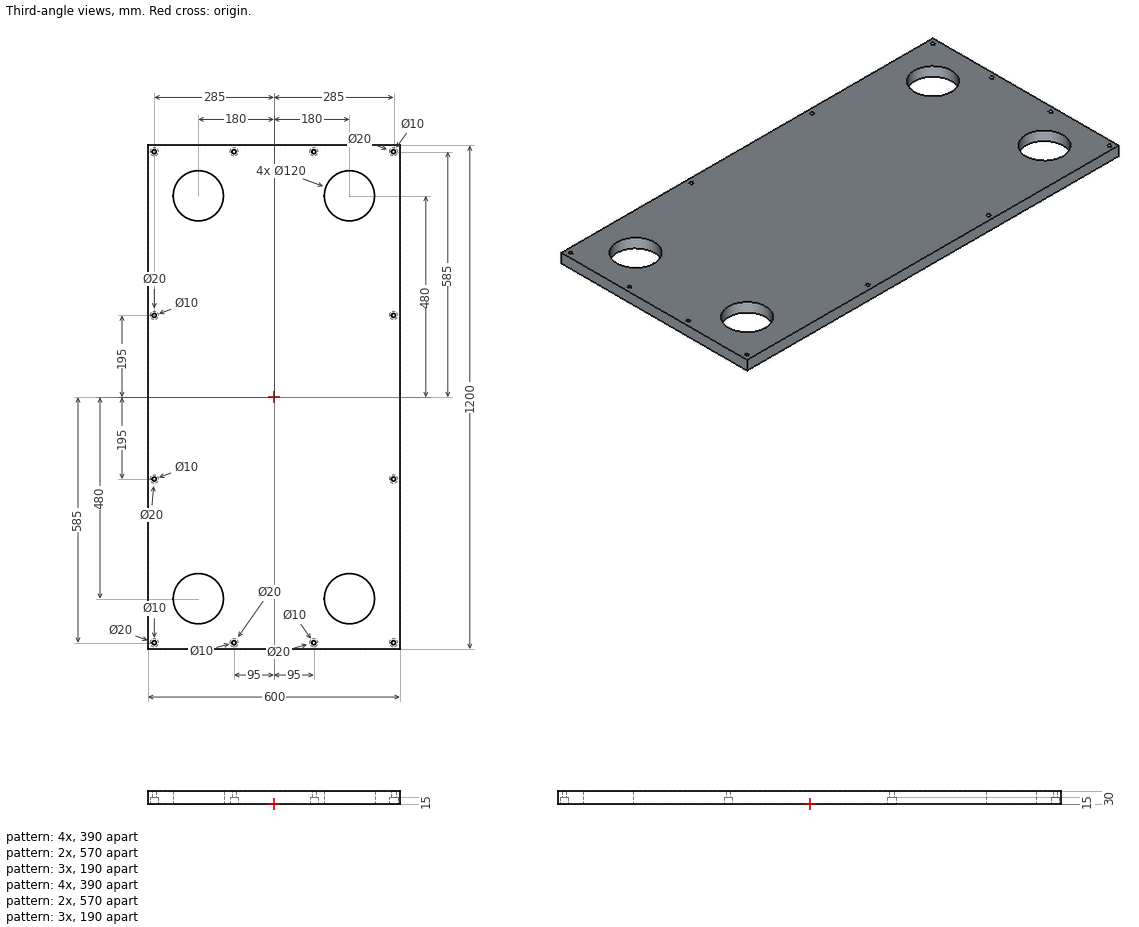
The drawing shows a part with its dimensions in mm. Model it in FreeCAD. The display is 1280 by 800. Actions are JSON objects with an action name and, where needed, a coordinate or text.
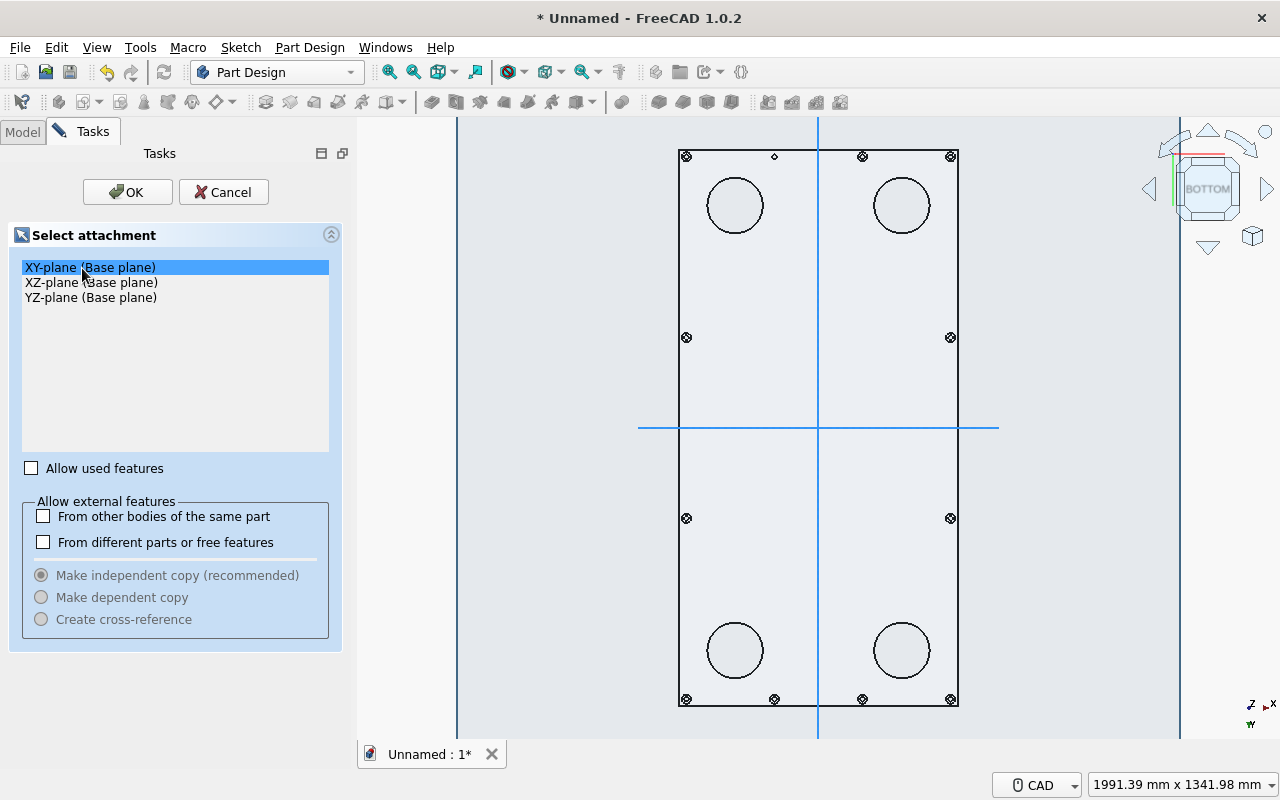
{"action": "left_click", "coordinate": [128, 192]}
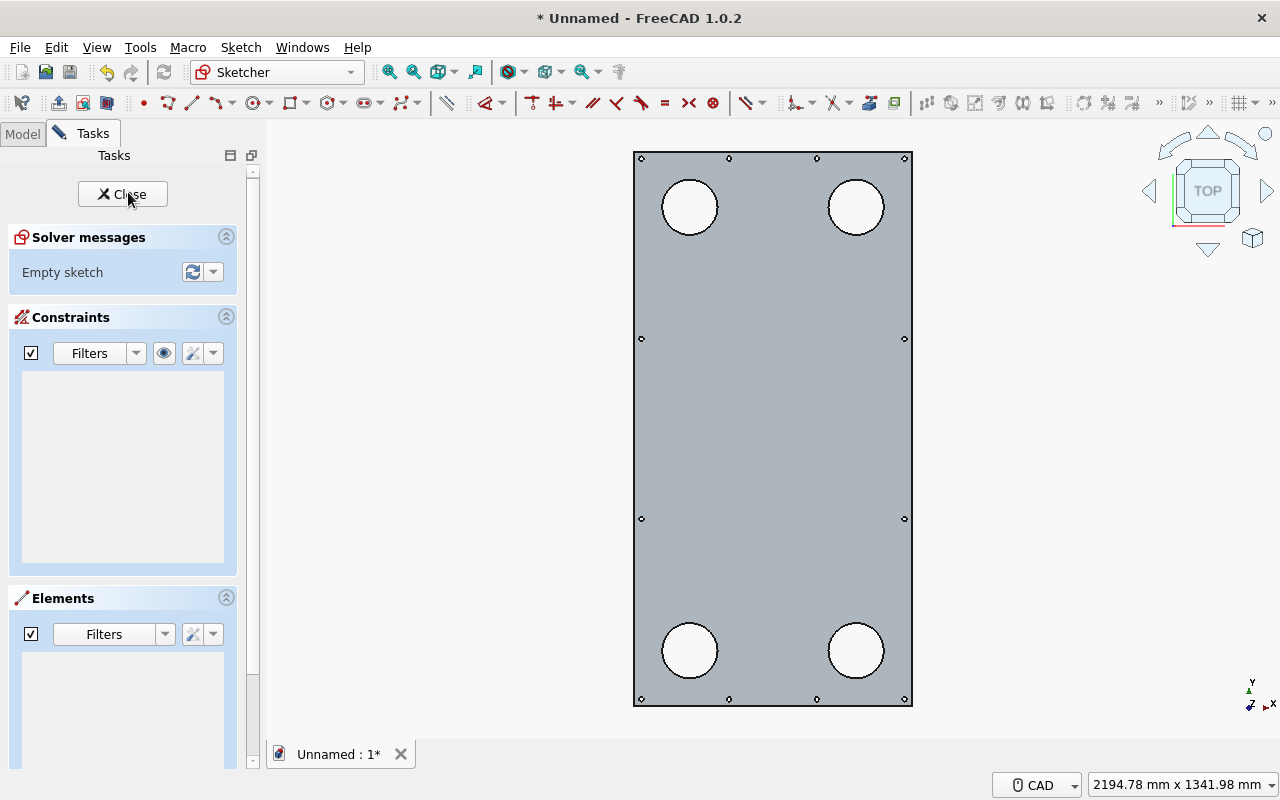
{"action": "left_click", "coordinate": [108, 104]}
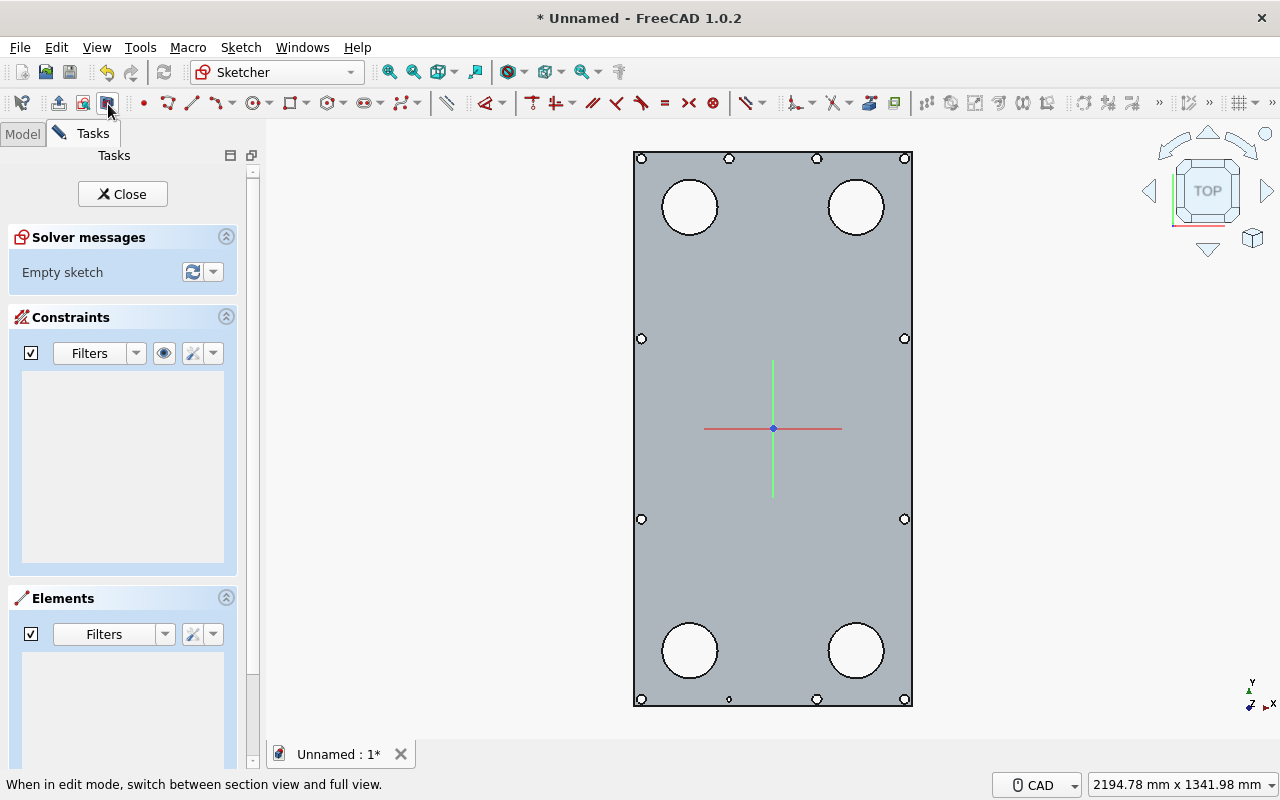
{"action": "scroll", "coordinate": [730, 711], "scroll_direction": "up", "scroll_amount": 15}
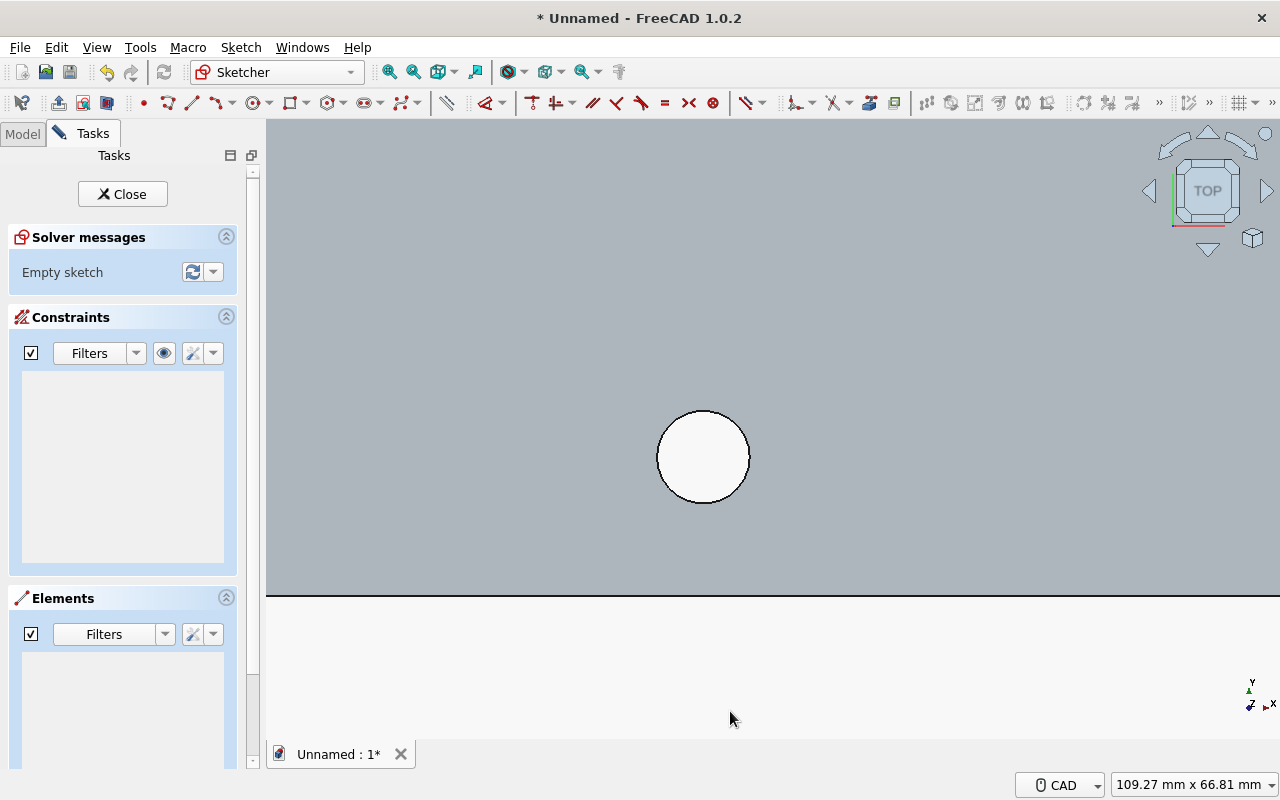
{"action": "scroll", "coordinate": [702, 480], "scroll_direction": "up", "scroll_amount": 4}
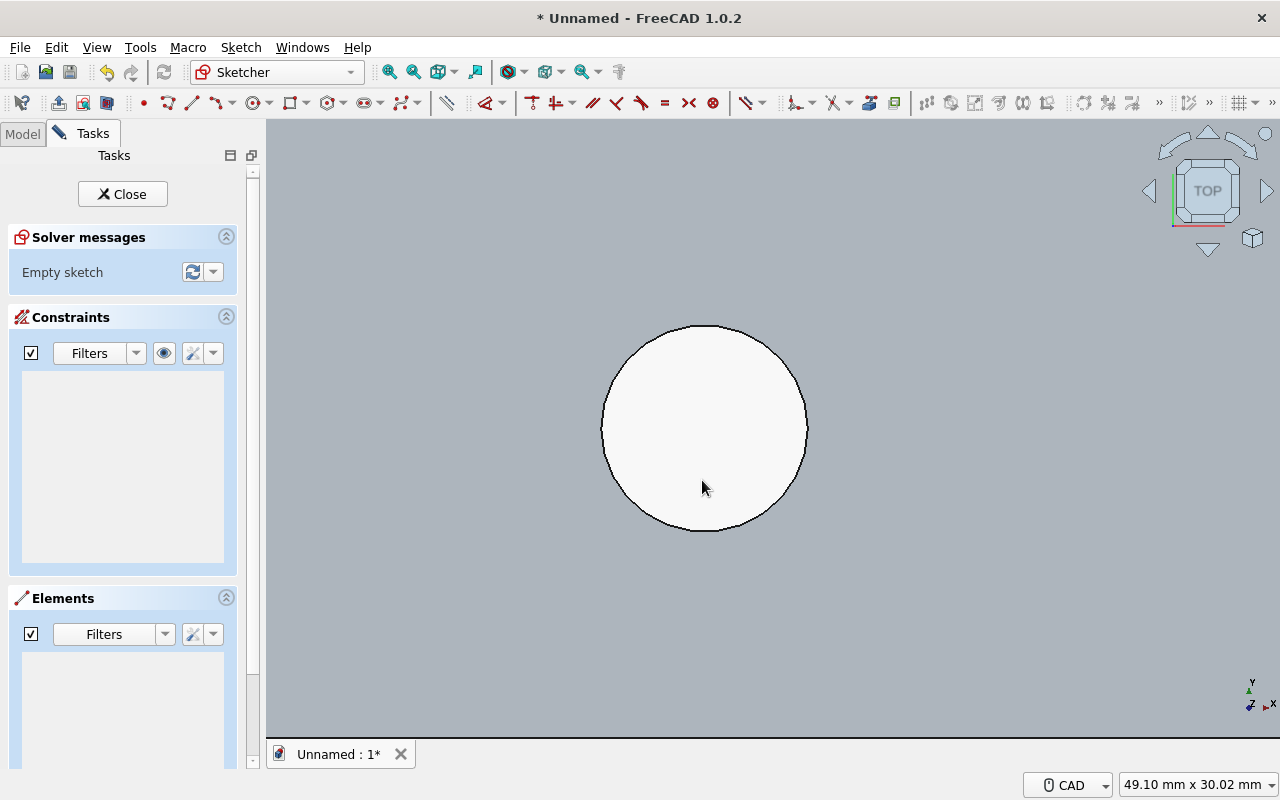
{"action": "left_click", "coordinate": [254, 104]}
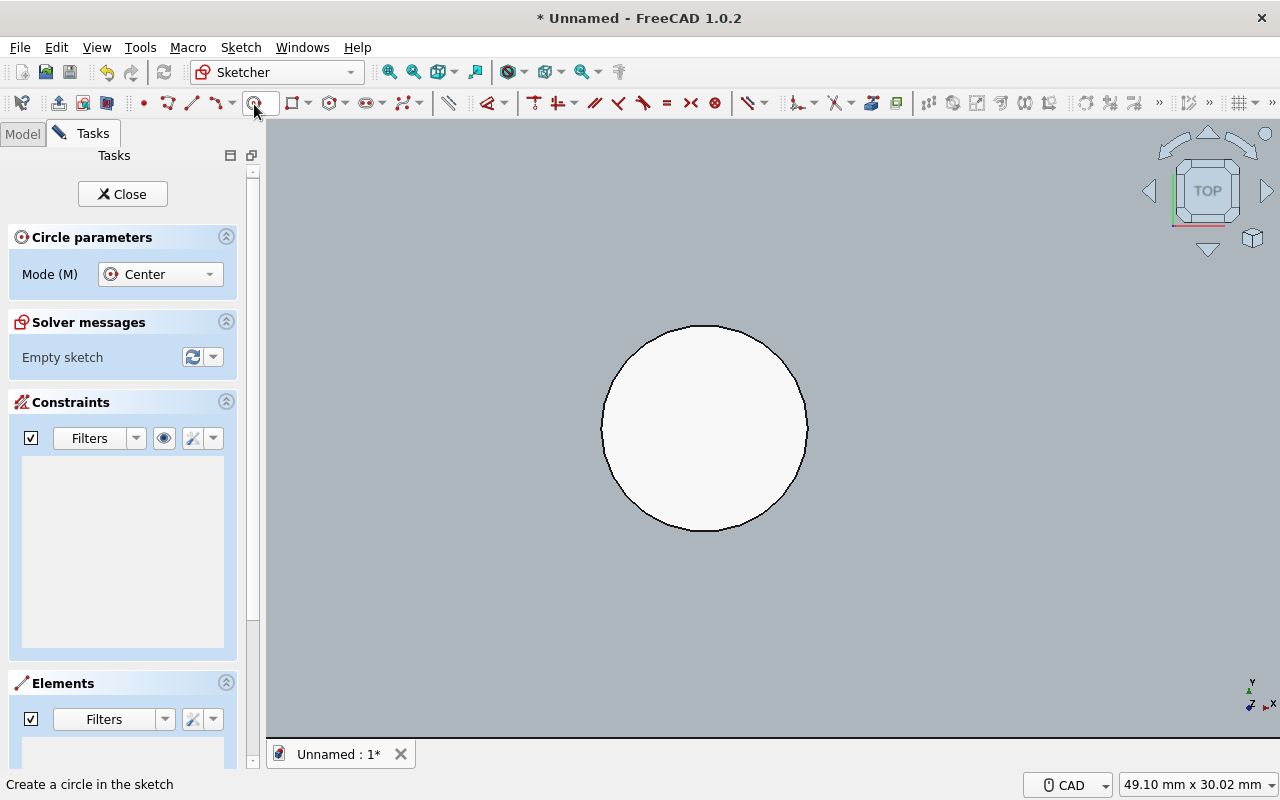
{"action": "left_click", "coordinate": [705, 429]}
{"action": "mouse_move", "coordinate": [851, 283]}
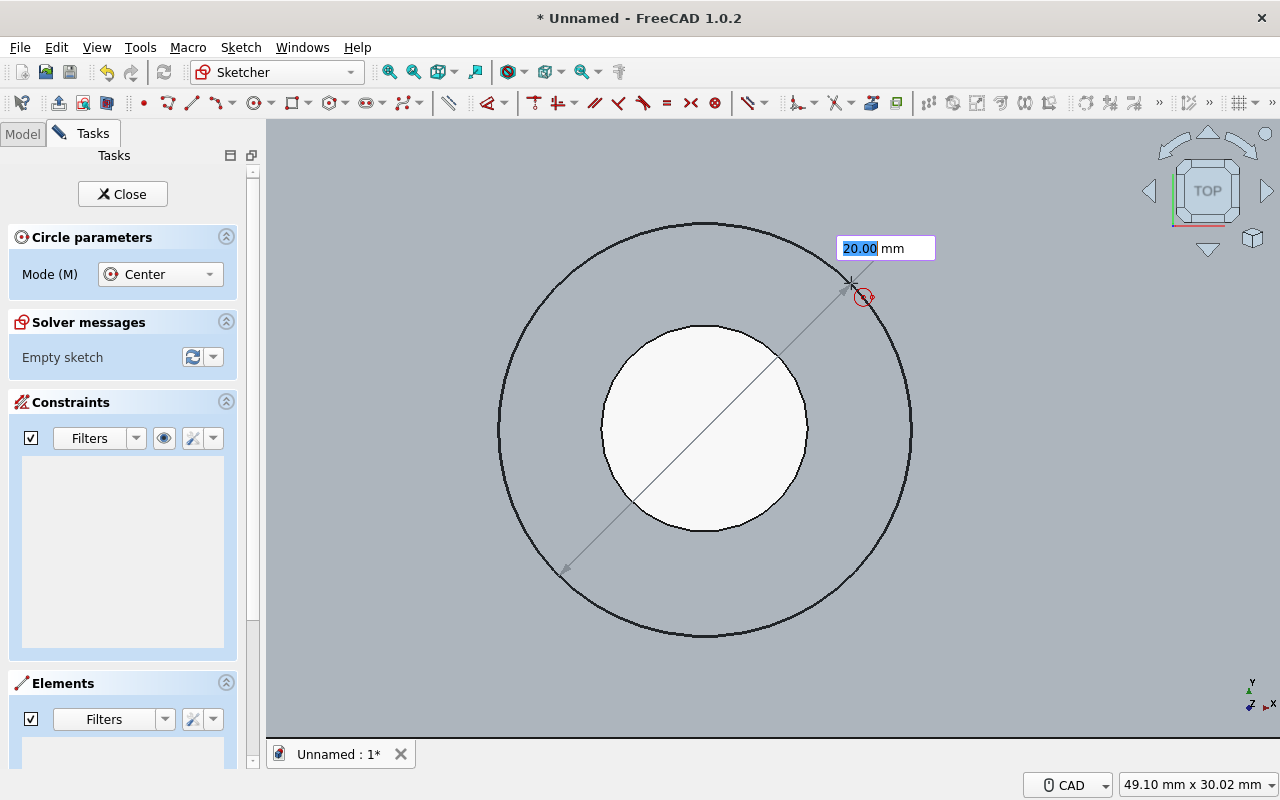
{"action": "type", "text": "20"}
{"action": "key", "text": "Return"}
{"action": "key", "text": "Escape"}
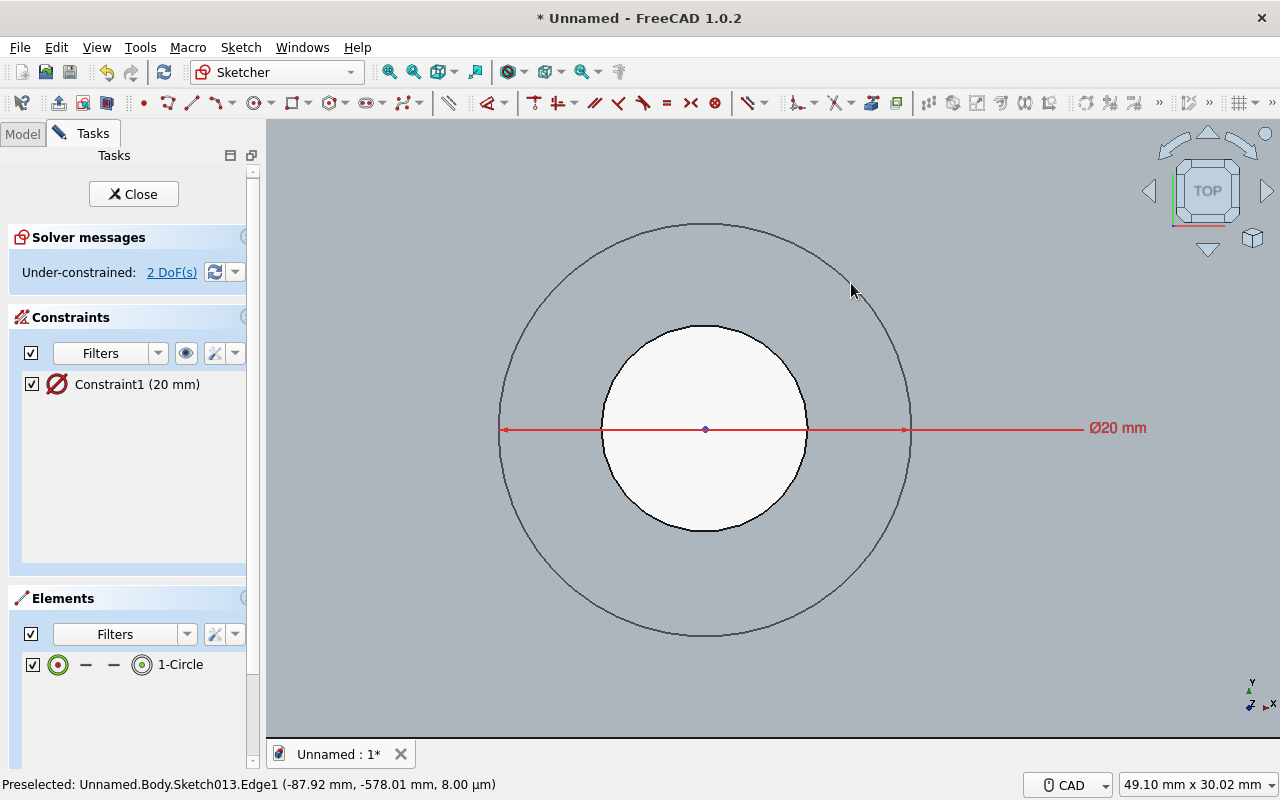
{"action": "left_click", "coordinate": [488, 104]}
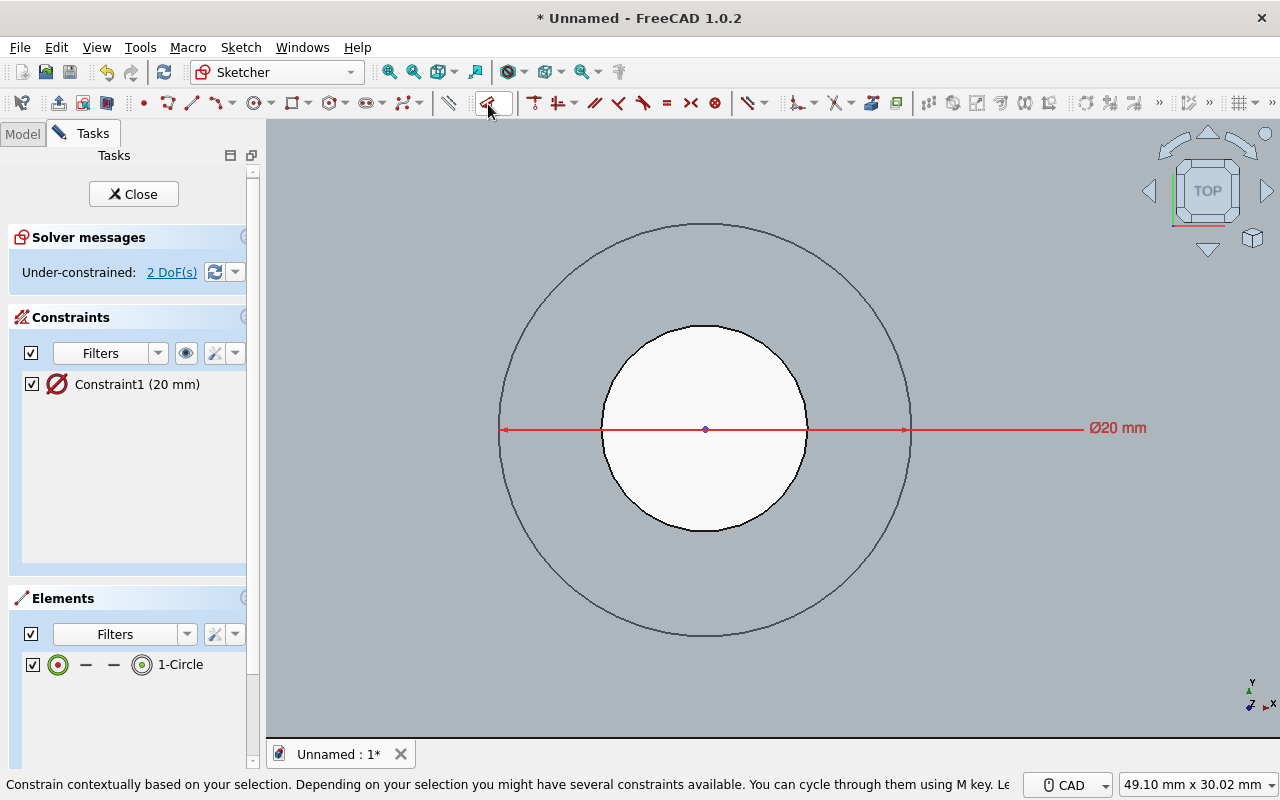
{"action": "left_click", "coordinate": [705, 430]}
{"action": "left_click", "coordinate": [816, 464]}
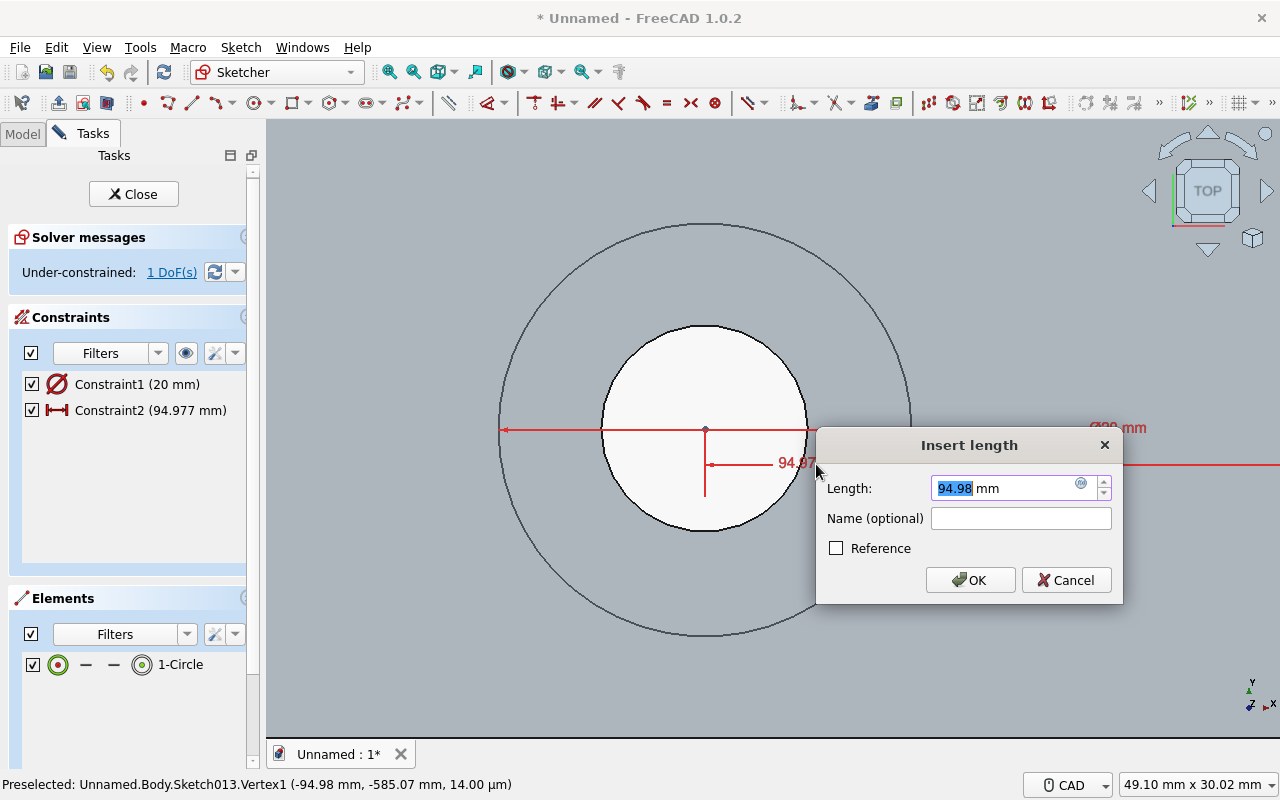
{"action": "type", "text": "95"}
{"action": "key", "text": "Return"}